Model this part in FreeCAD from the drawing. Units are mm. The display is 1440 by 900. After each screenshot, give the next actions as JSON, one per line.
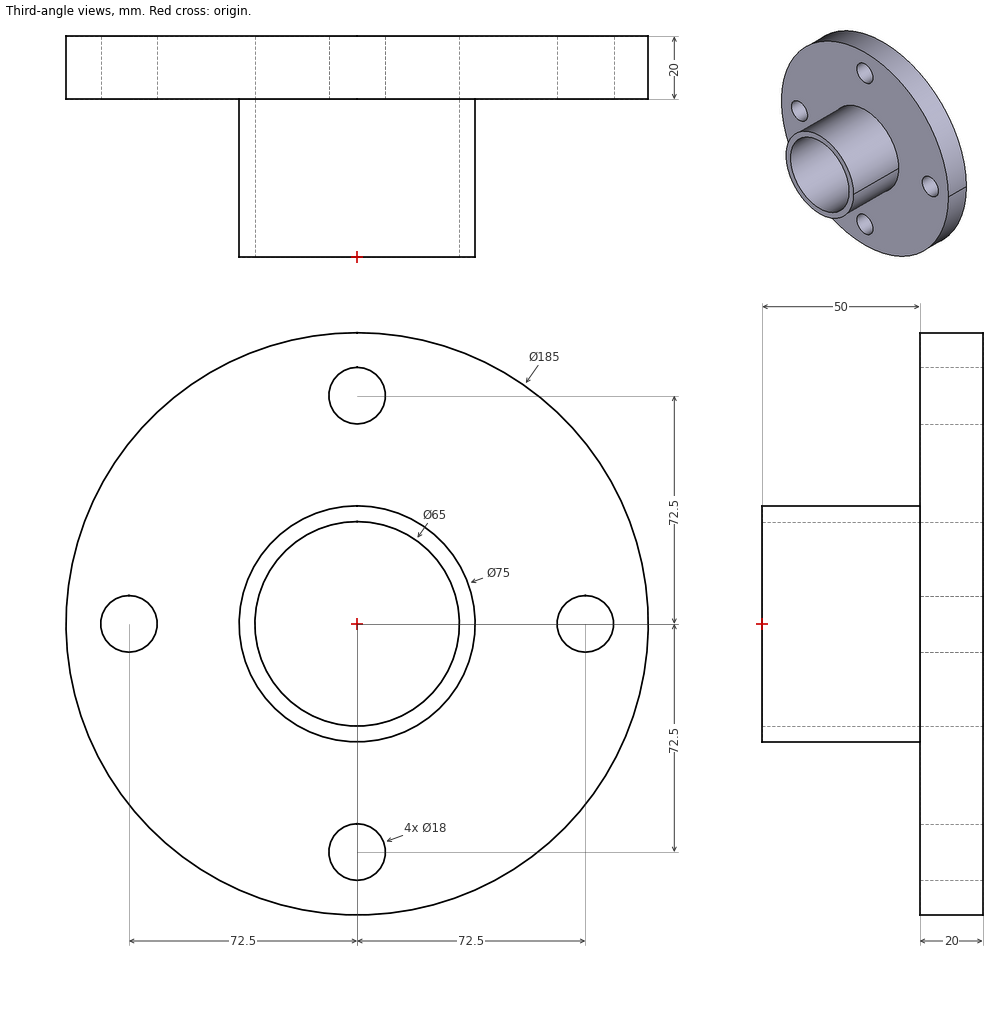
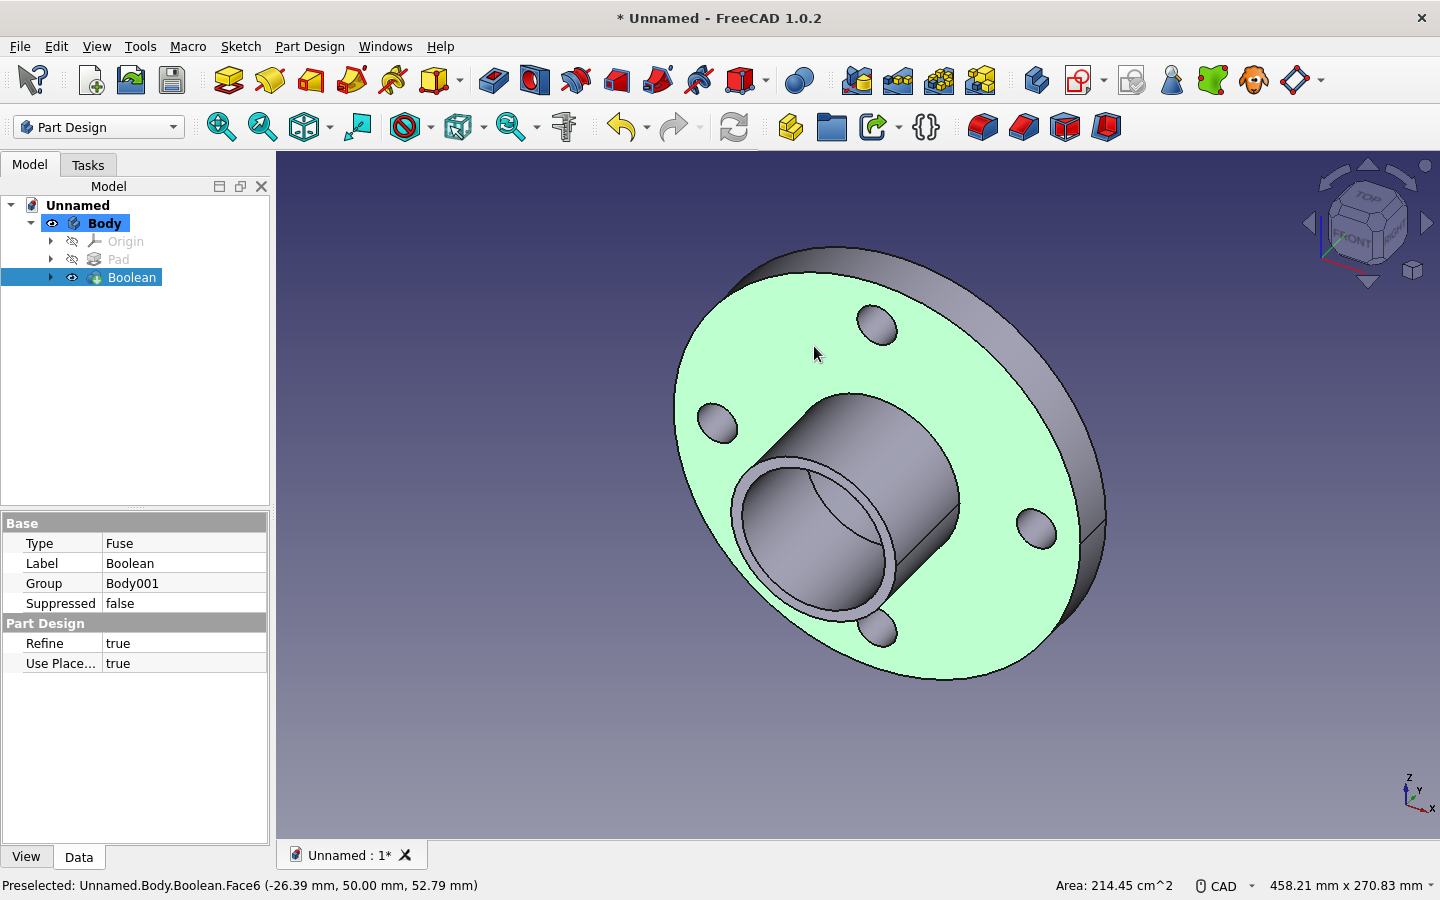
{"action": "left_click", "coordinate": [1078, 80]}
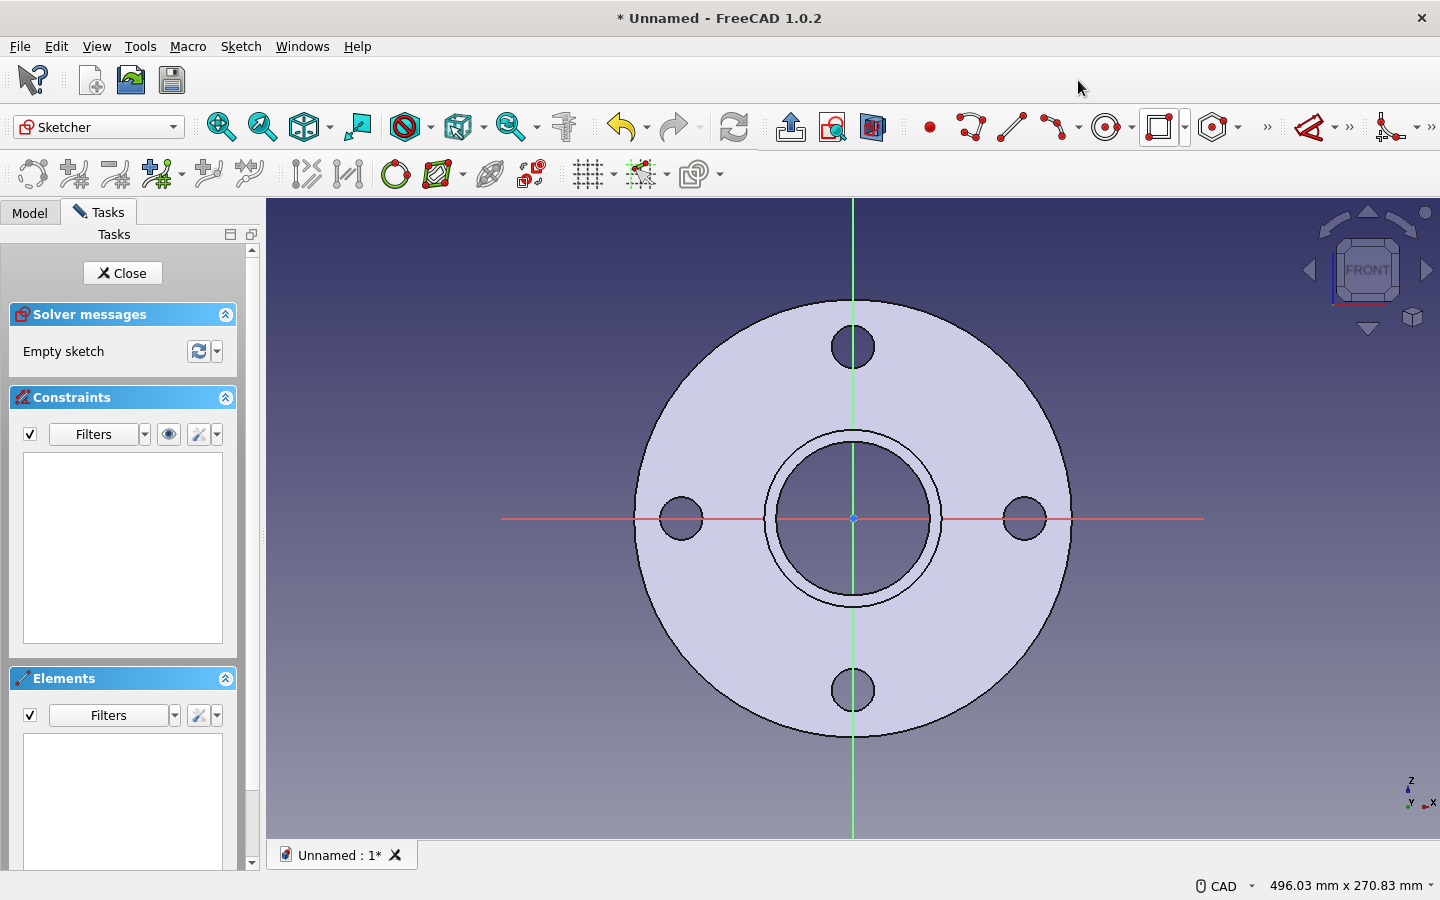
{"action": "scroll", "coordinate": [909, 518], "scroll_direction": "up", "scroll_amount": 4}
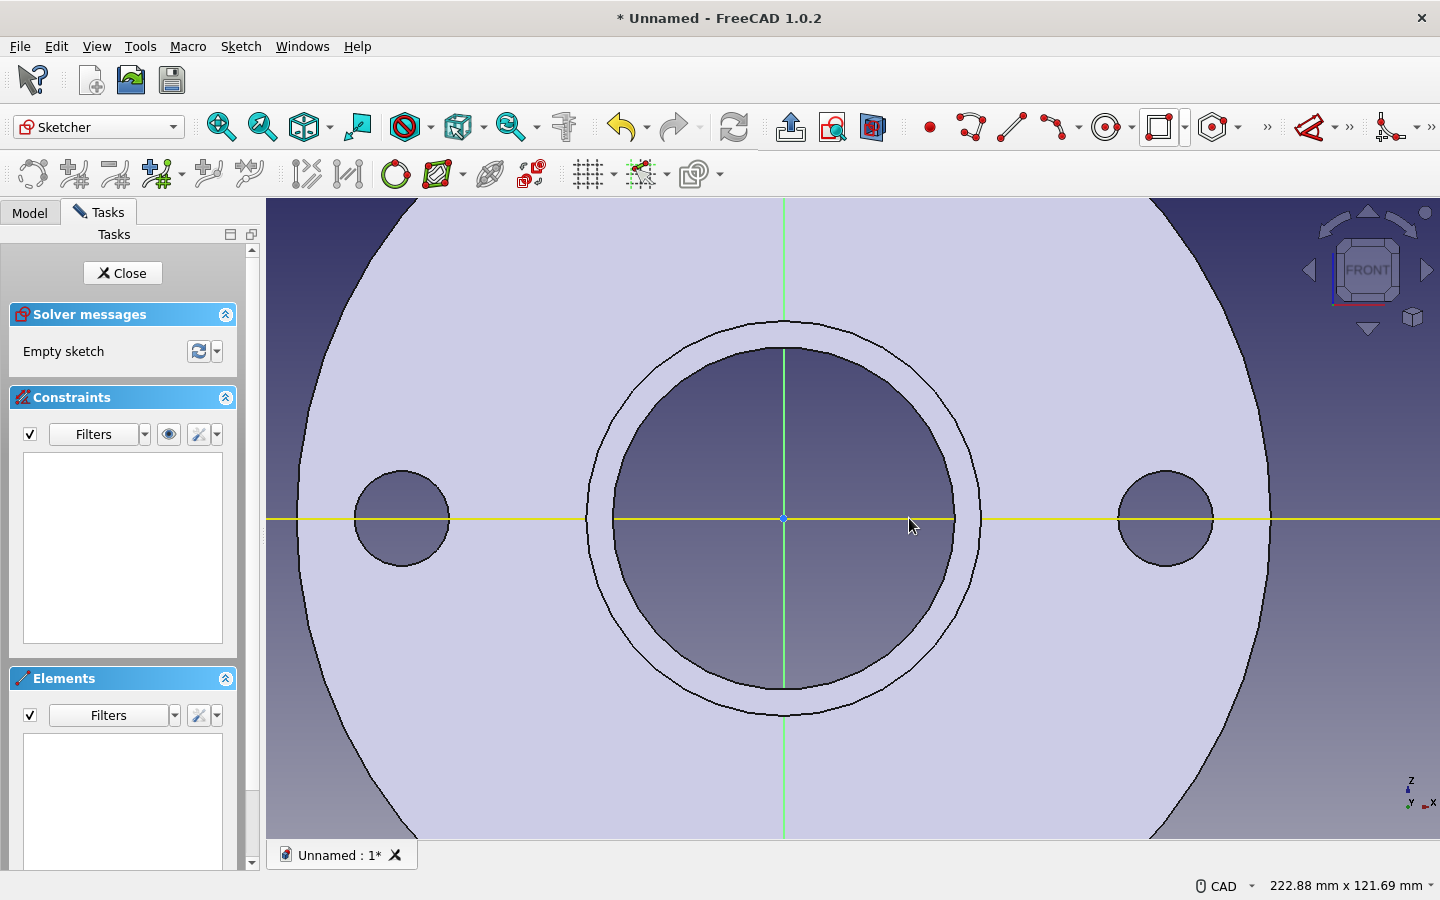
{"action": "key", "text": "g c"}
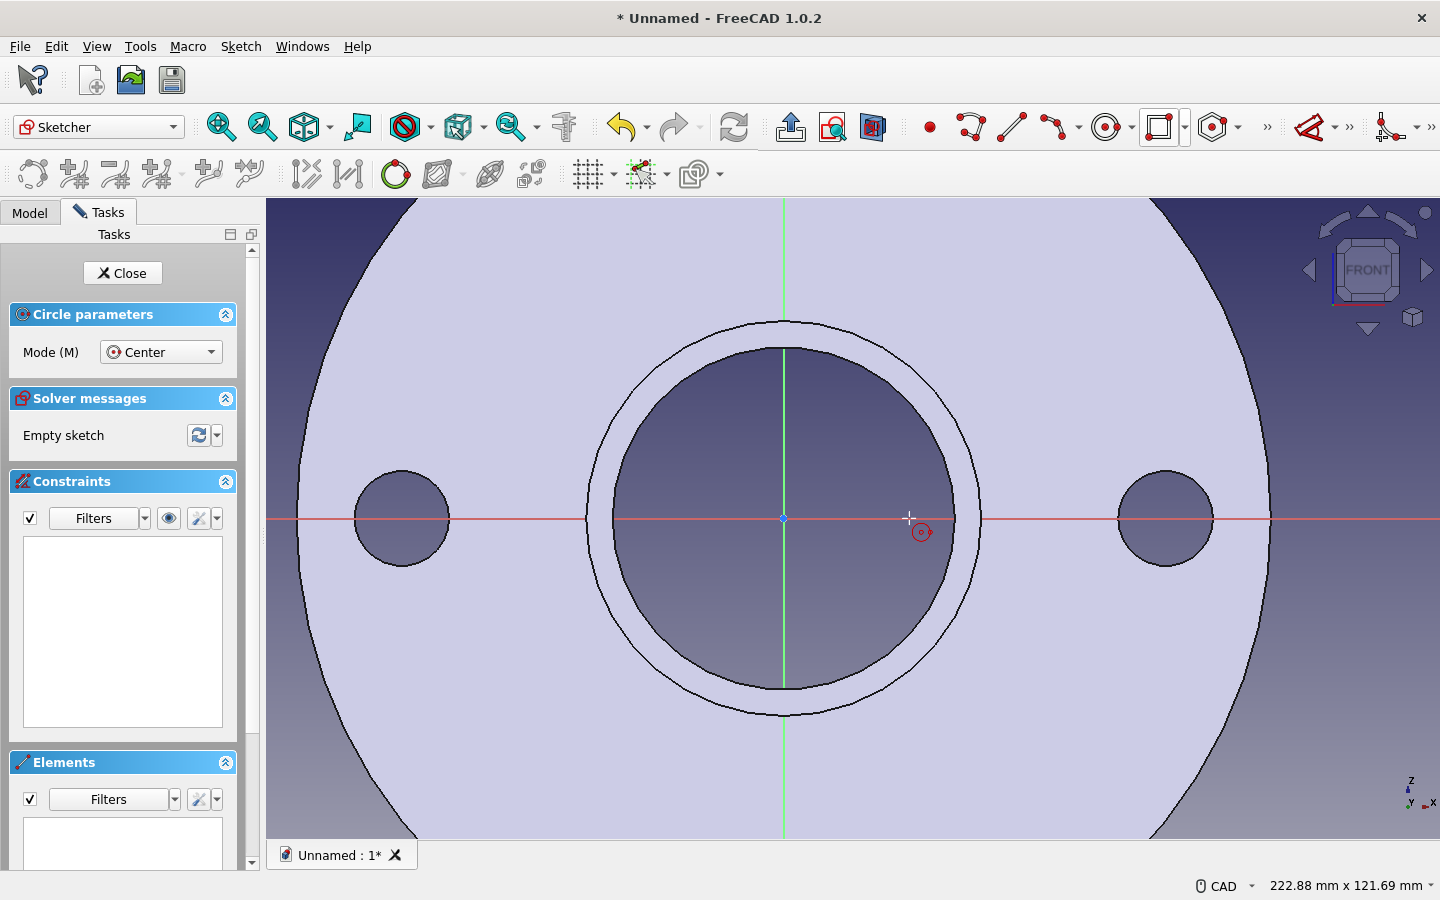
{"action": "left_click", "coordinate": [784, 518]}
{"action": "left_click", "coordinate": [923, 379]}
{"action": "key", "text": "Escape"}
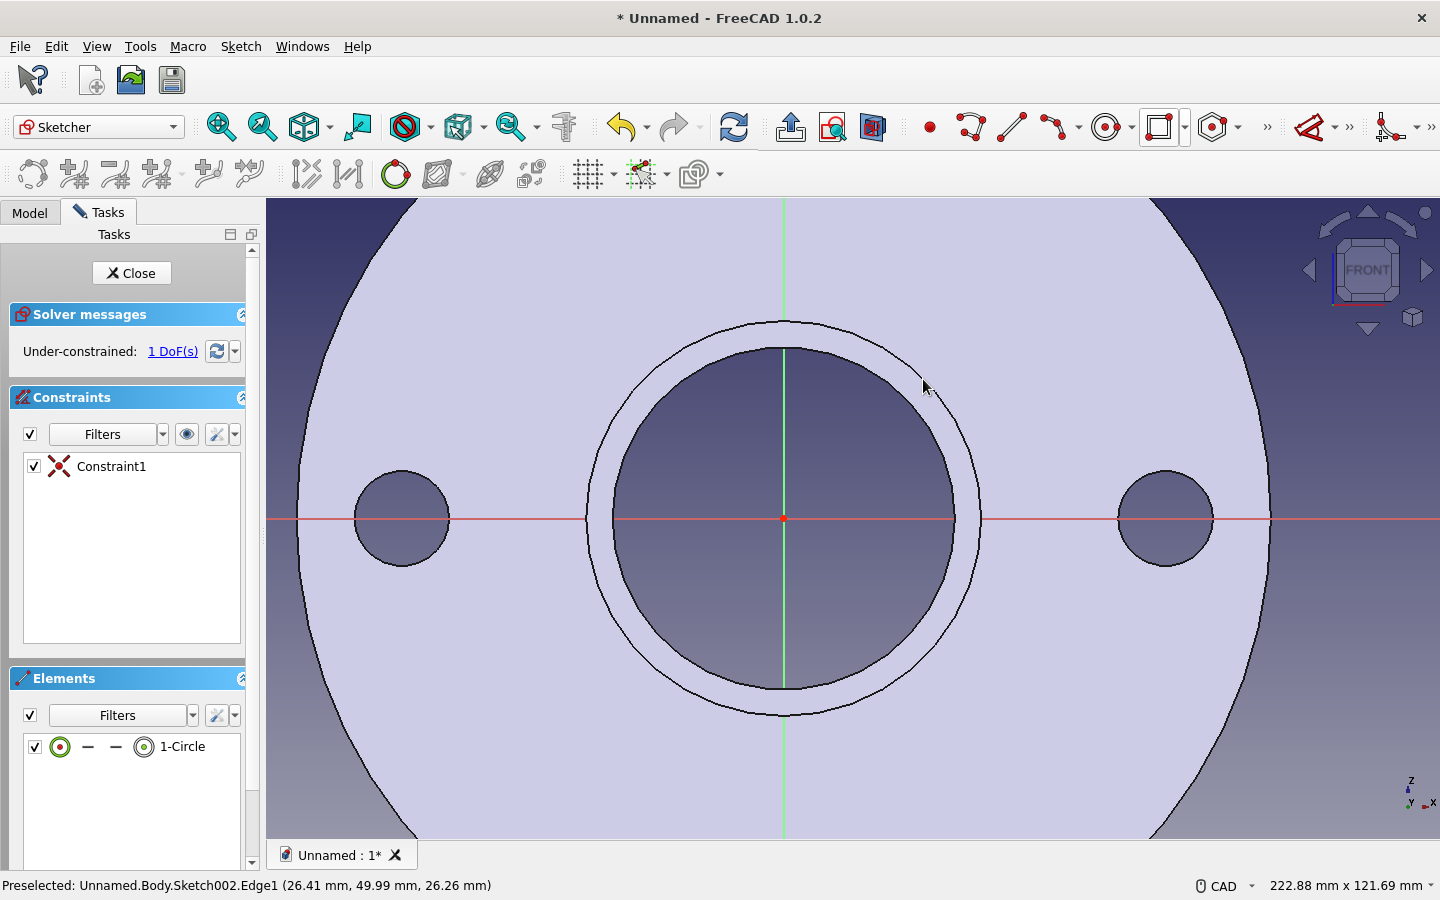
{"action": "key", "text": "d"}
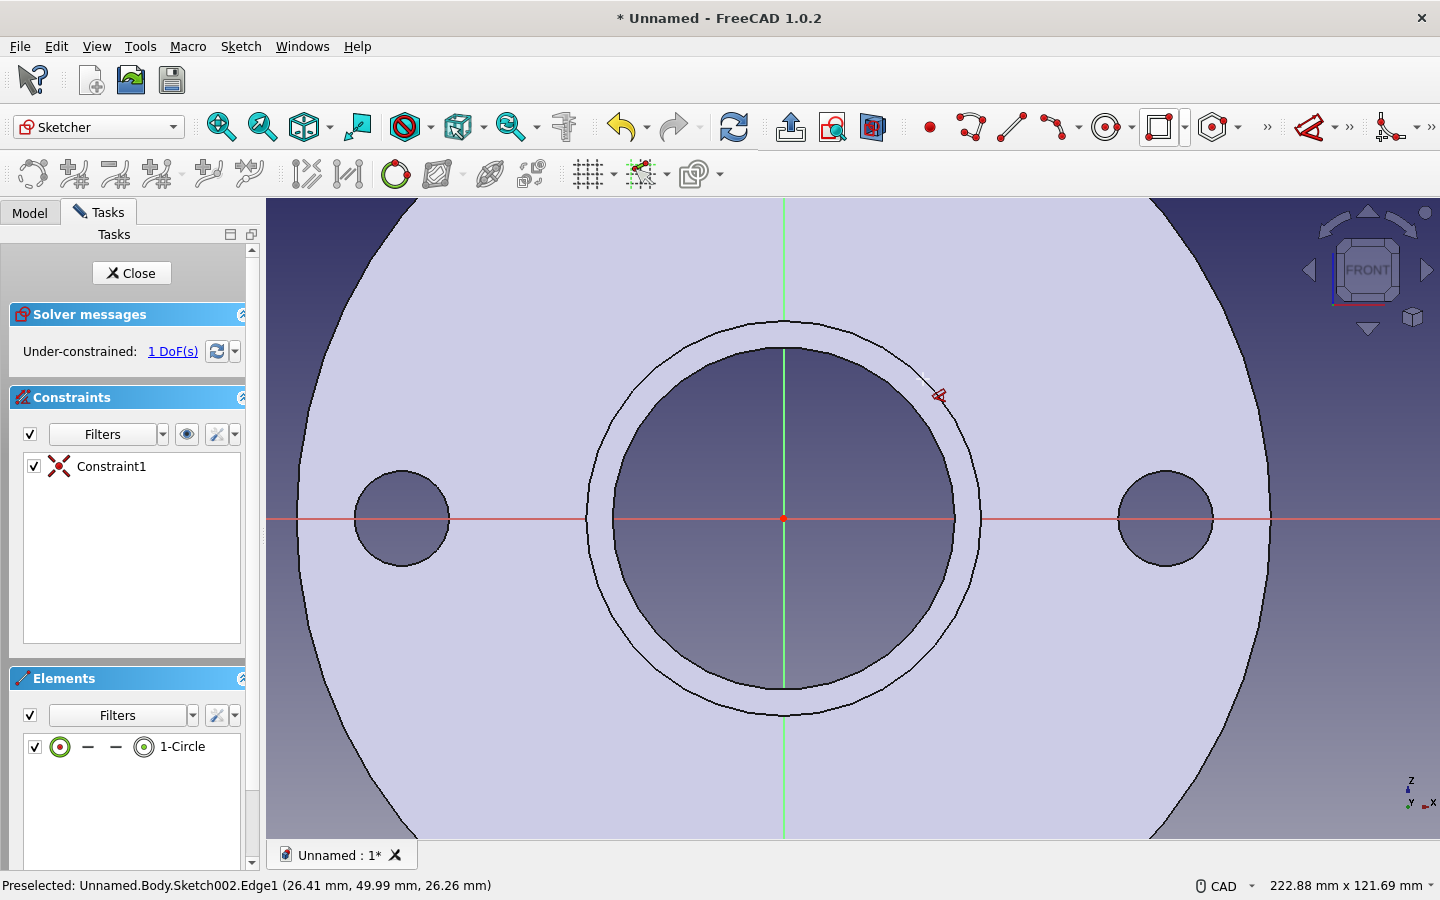
{"action": "left_click", "coordinate": [922, 379]}
{"action": "left_click", "coordinate": [945, 356]}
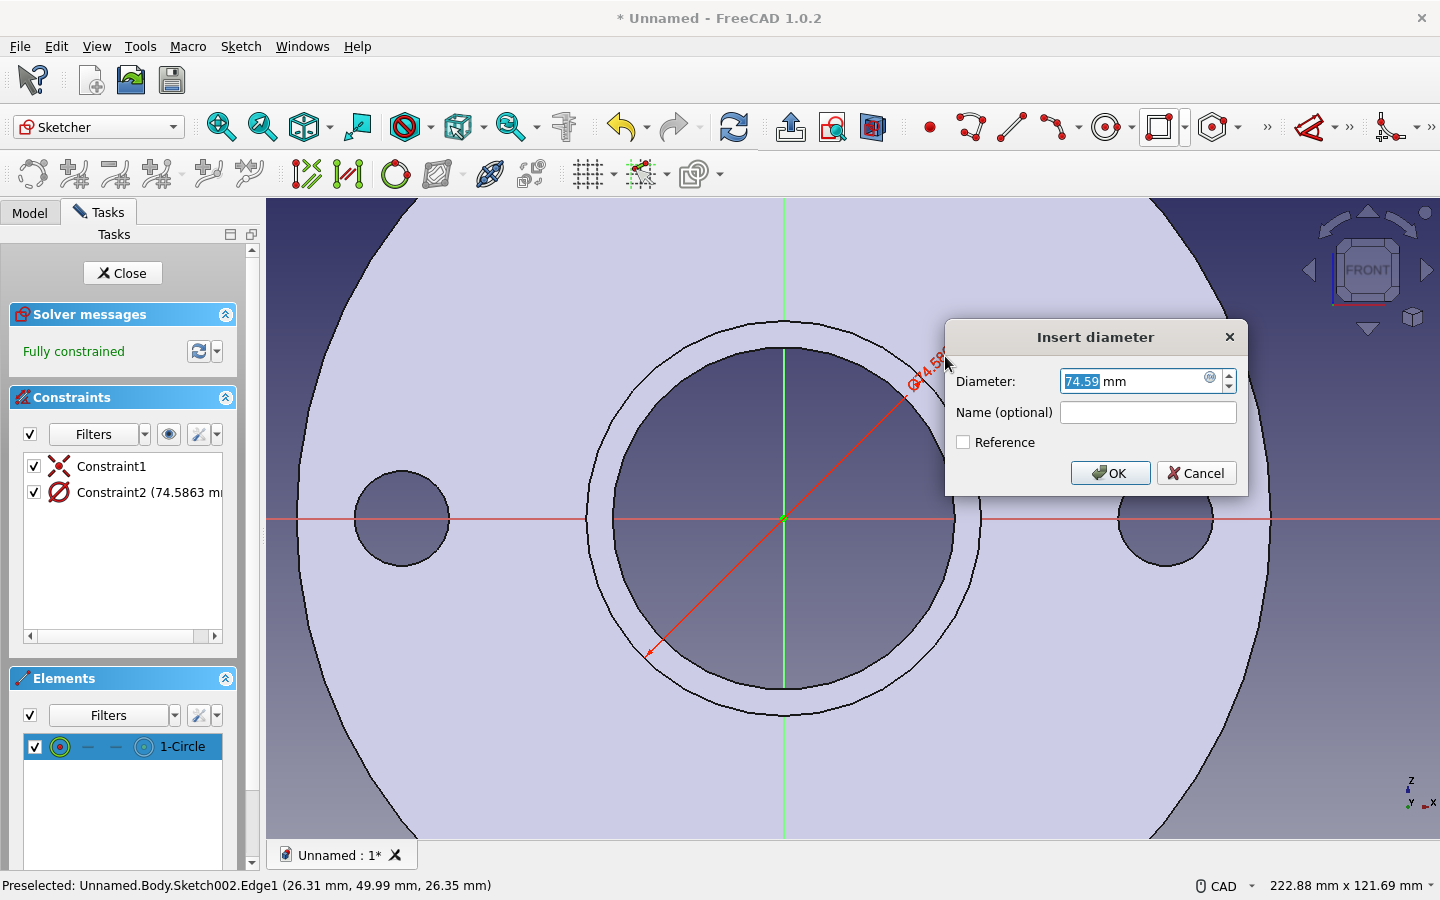
{"action": "type", "text": "75"}
{"action": "key", "text": "Return"}
{"action": "key", "text": "Escape"}